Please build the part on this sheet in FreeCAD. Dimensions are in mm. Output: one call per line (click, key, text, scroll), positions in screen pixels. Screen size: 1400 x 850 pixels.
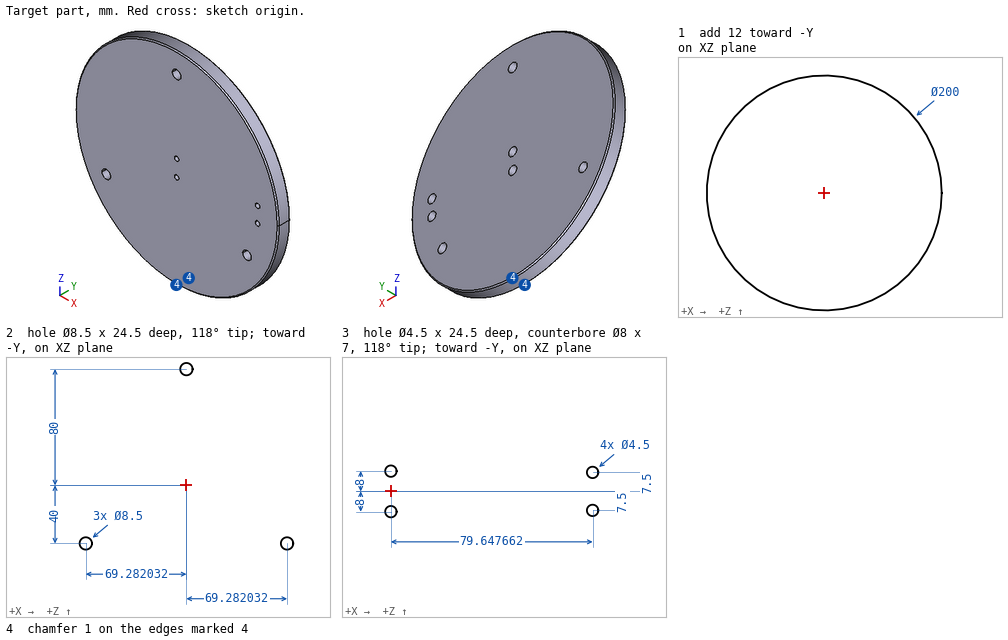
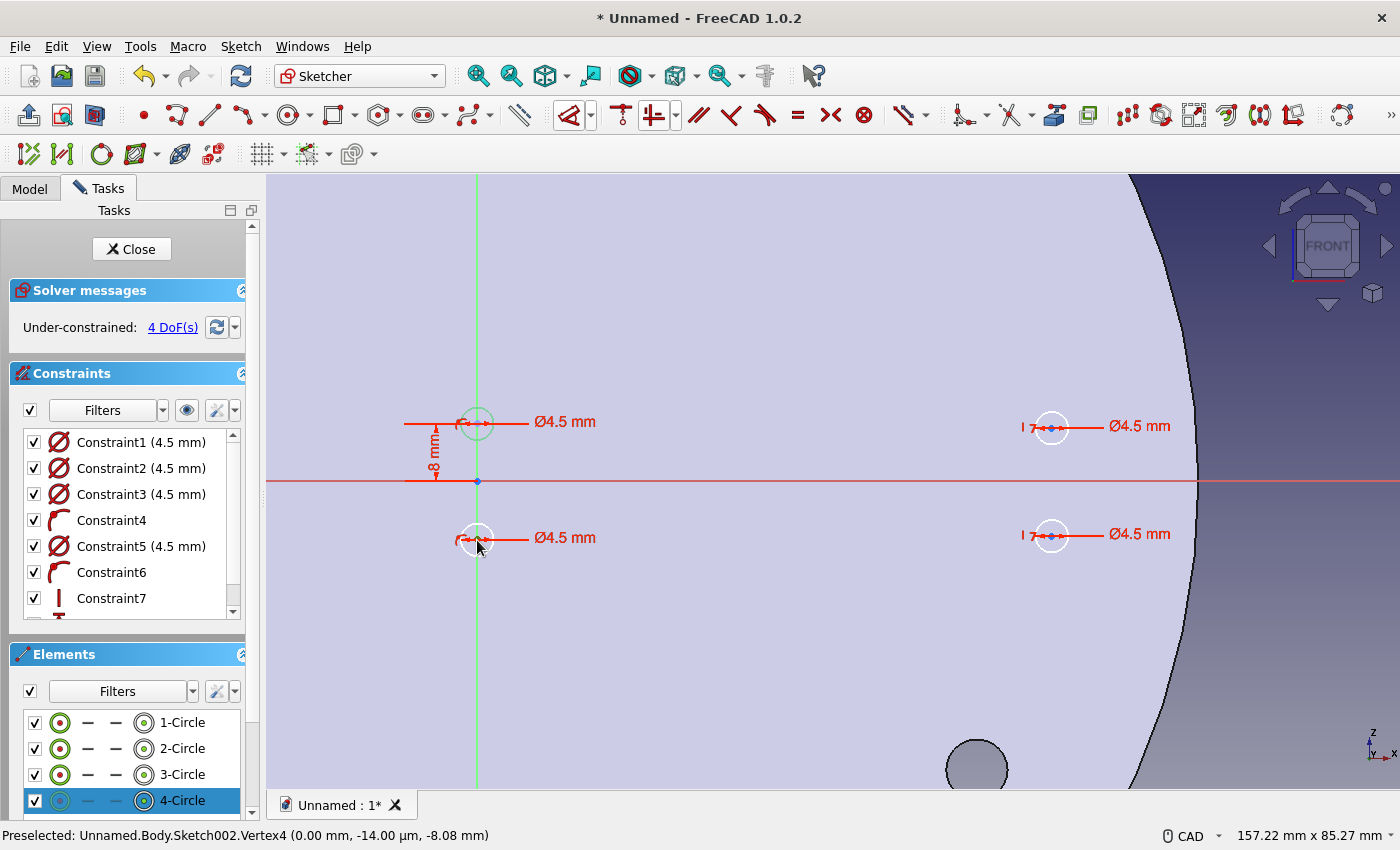
key(i)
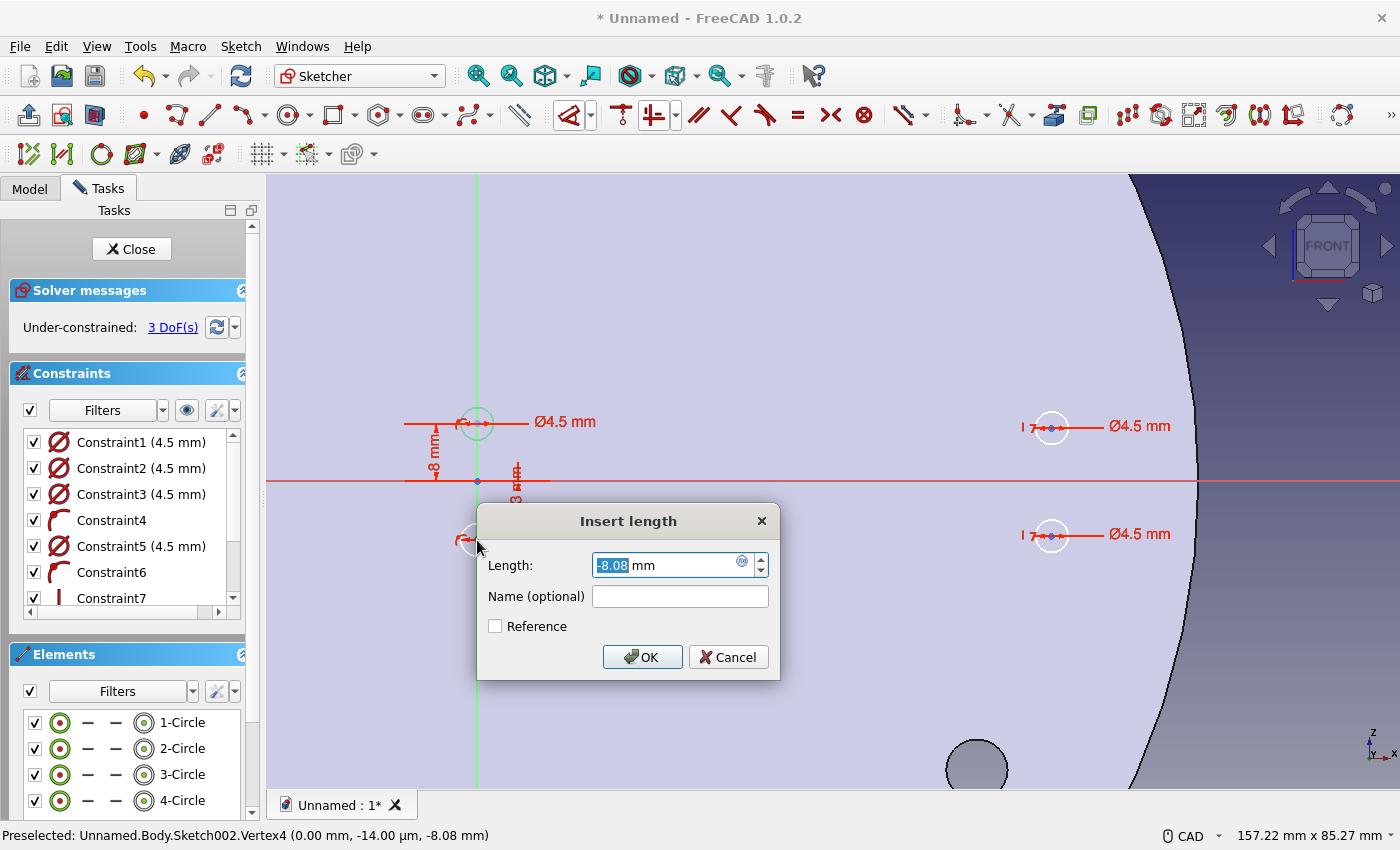
text(-8)
key(Return)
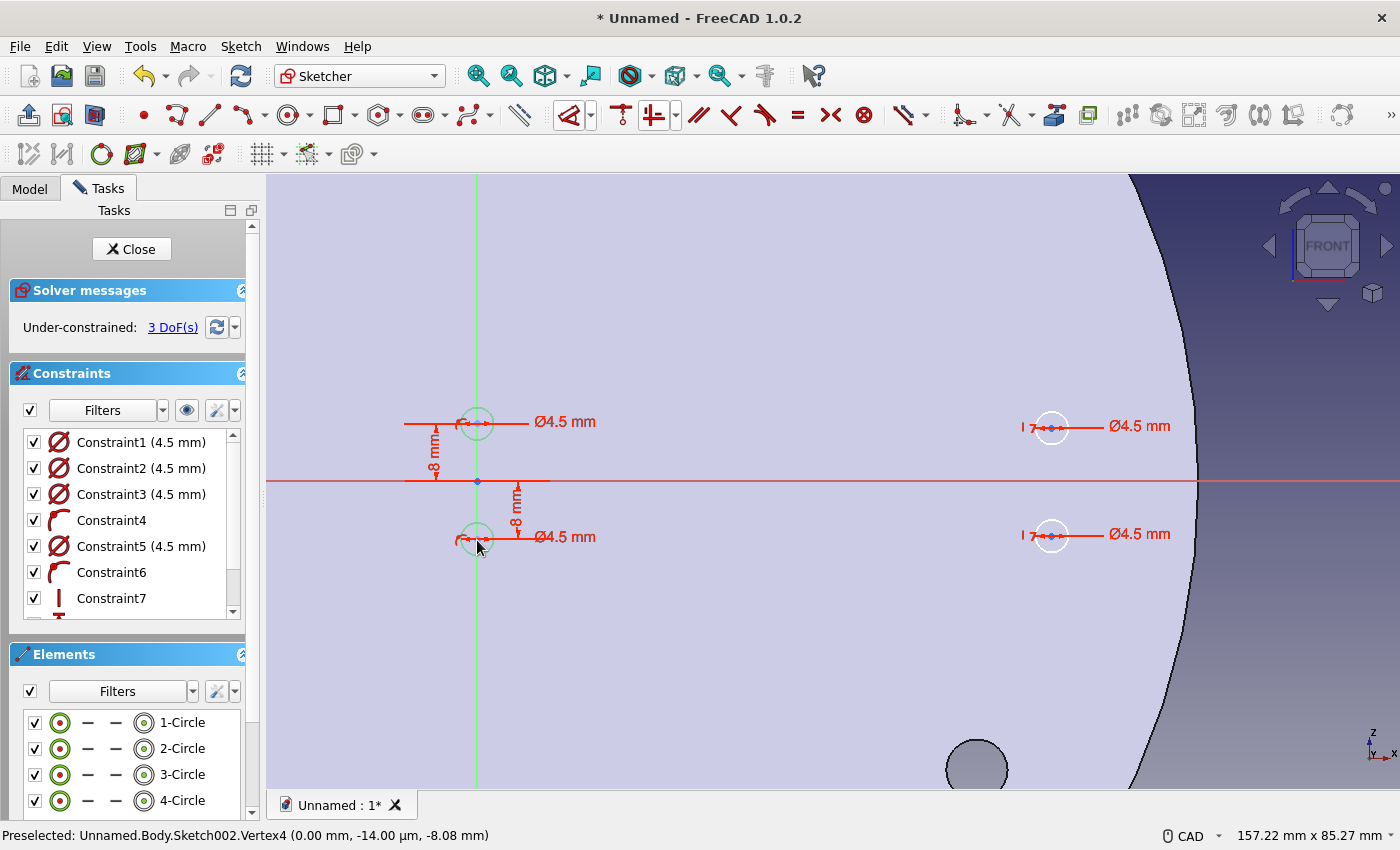
click(1052, 536)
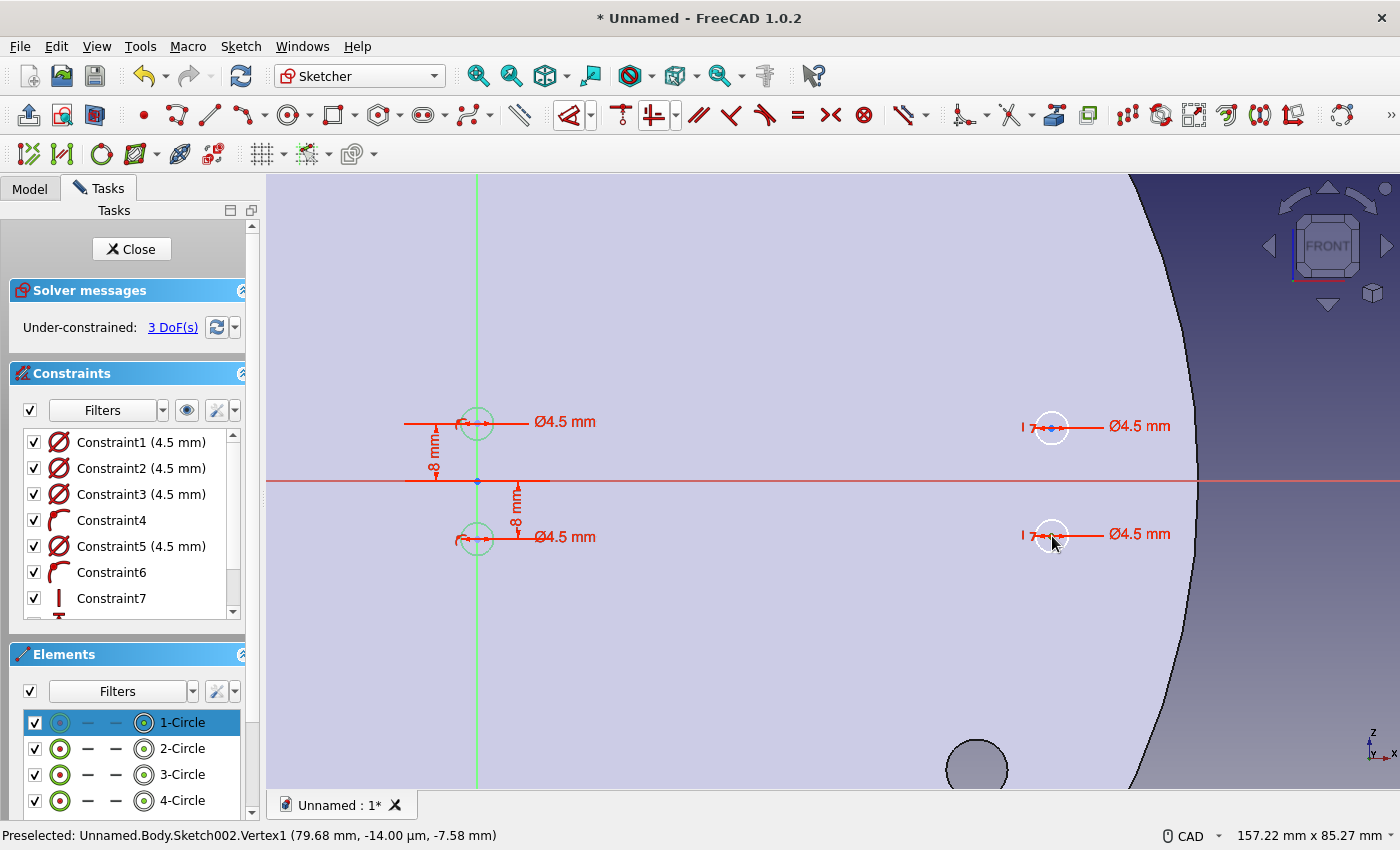
key(i)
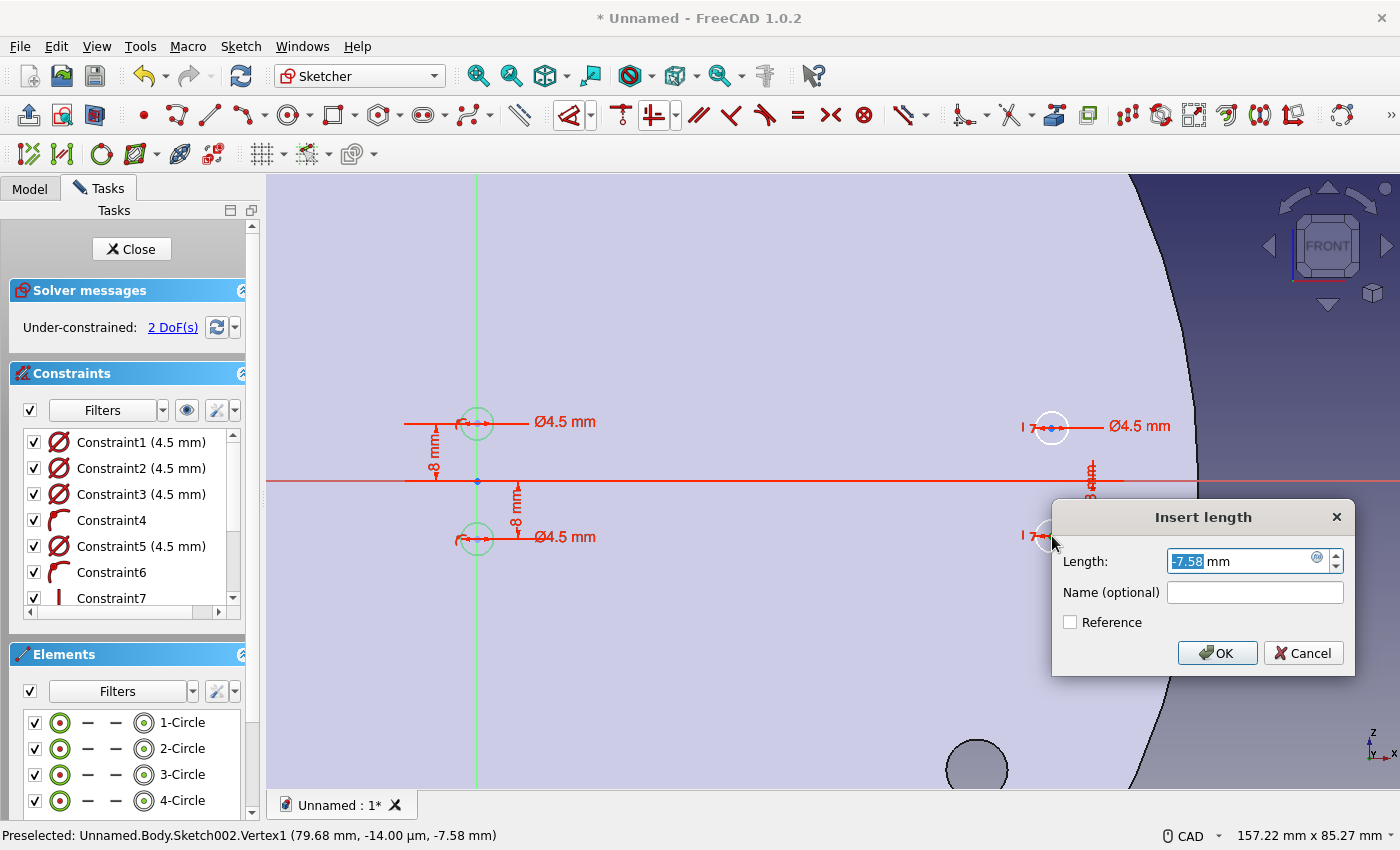
text(-7.5)
key(Return)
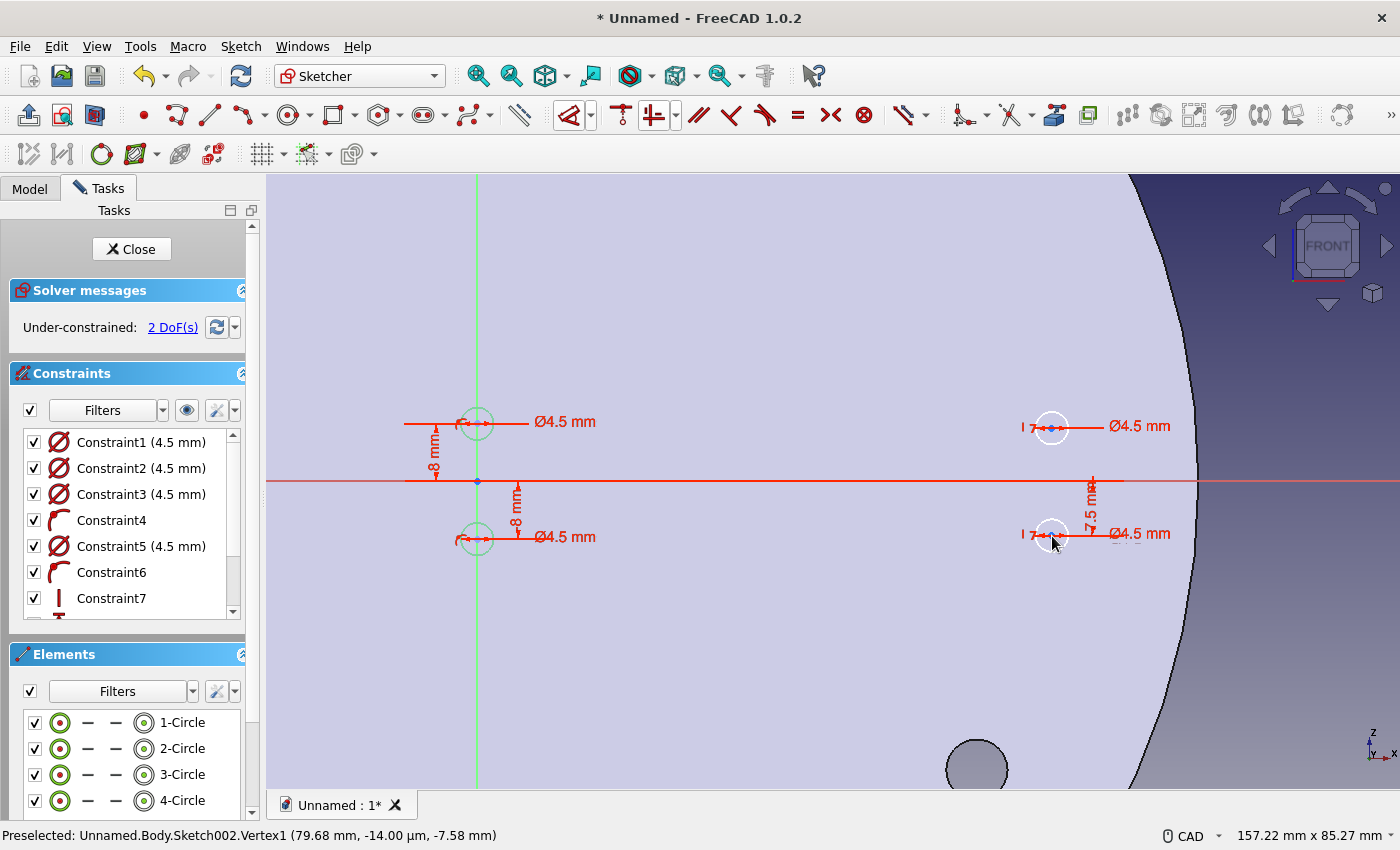
click(1052, 428)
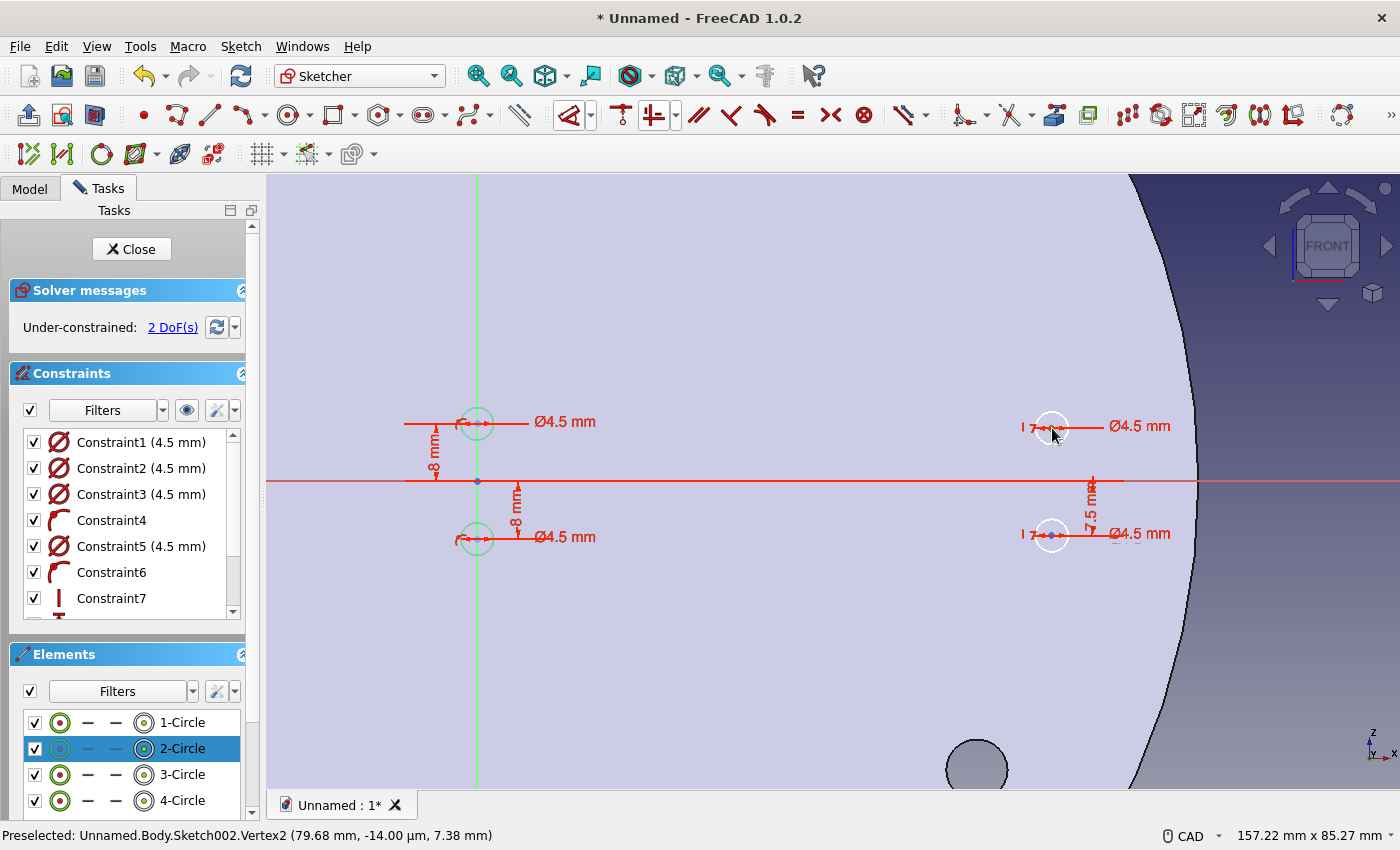
click(590, 116)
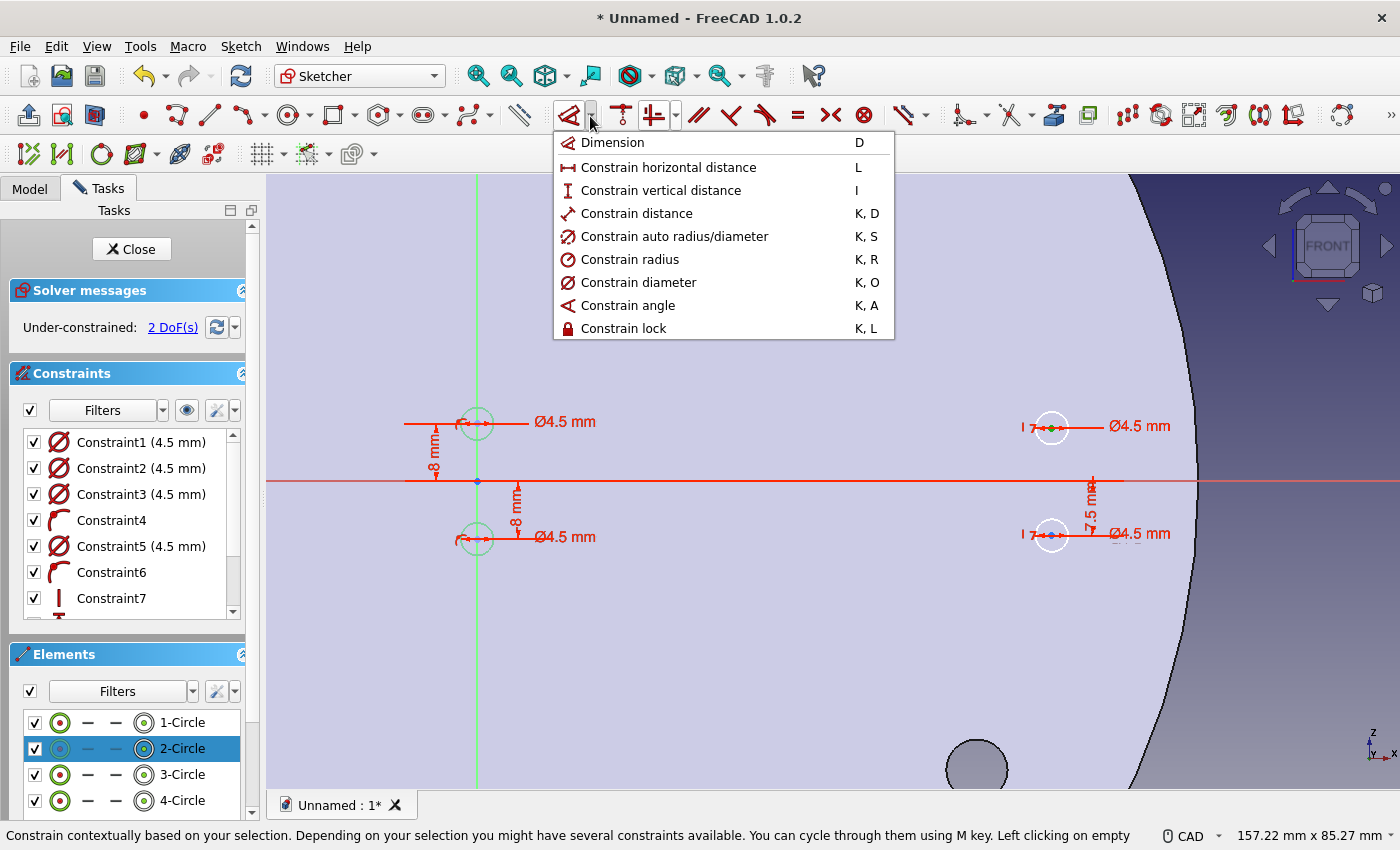
click(724, 190)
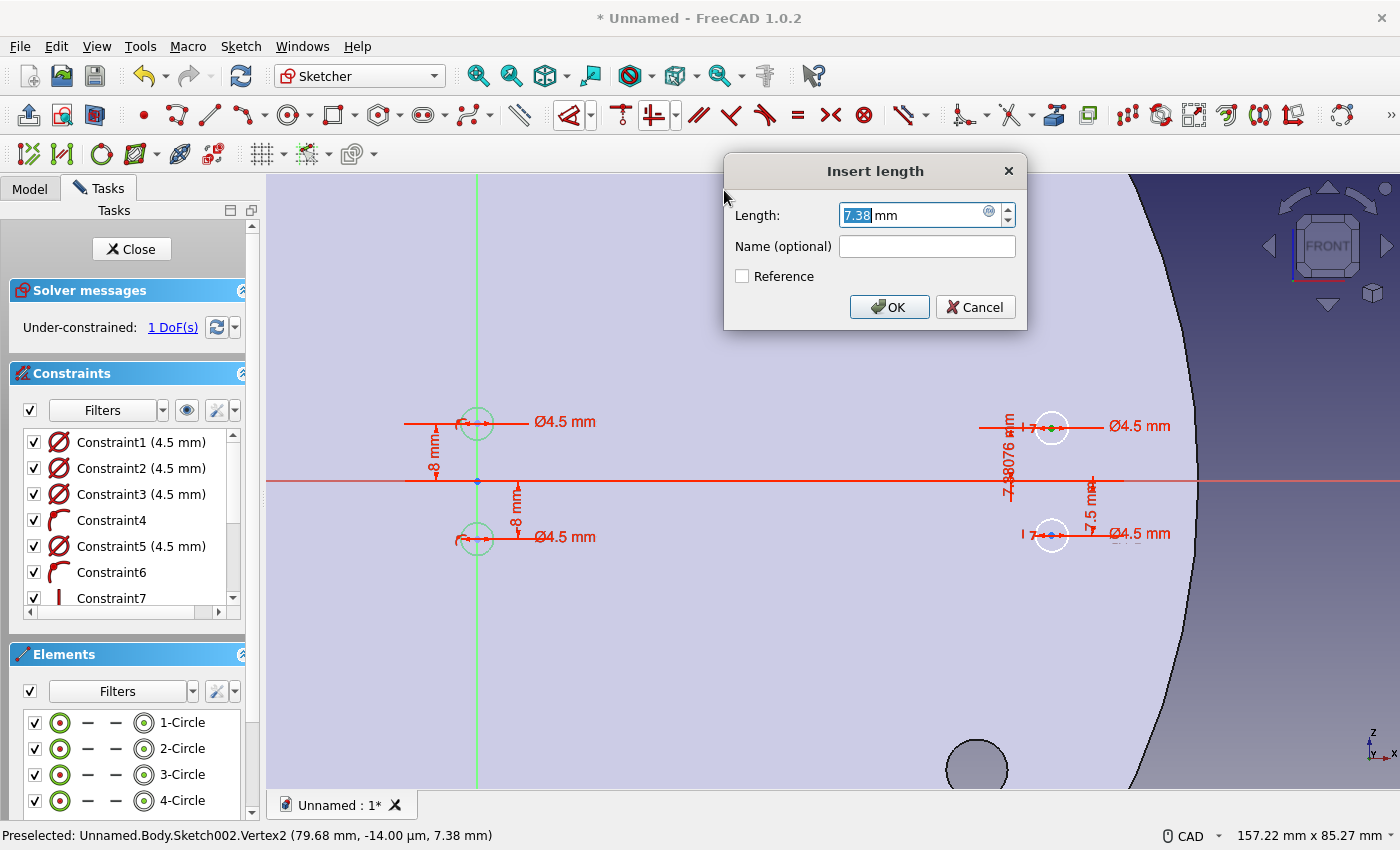
text(7.5)
key(Return)